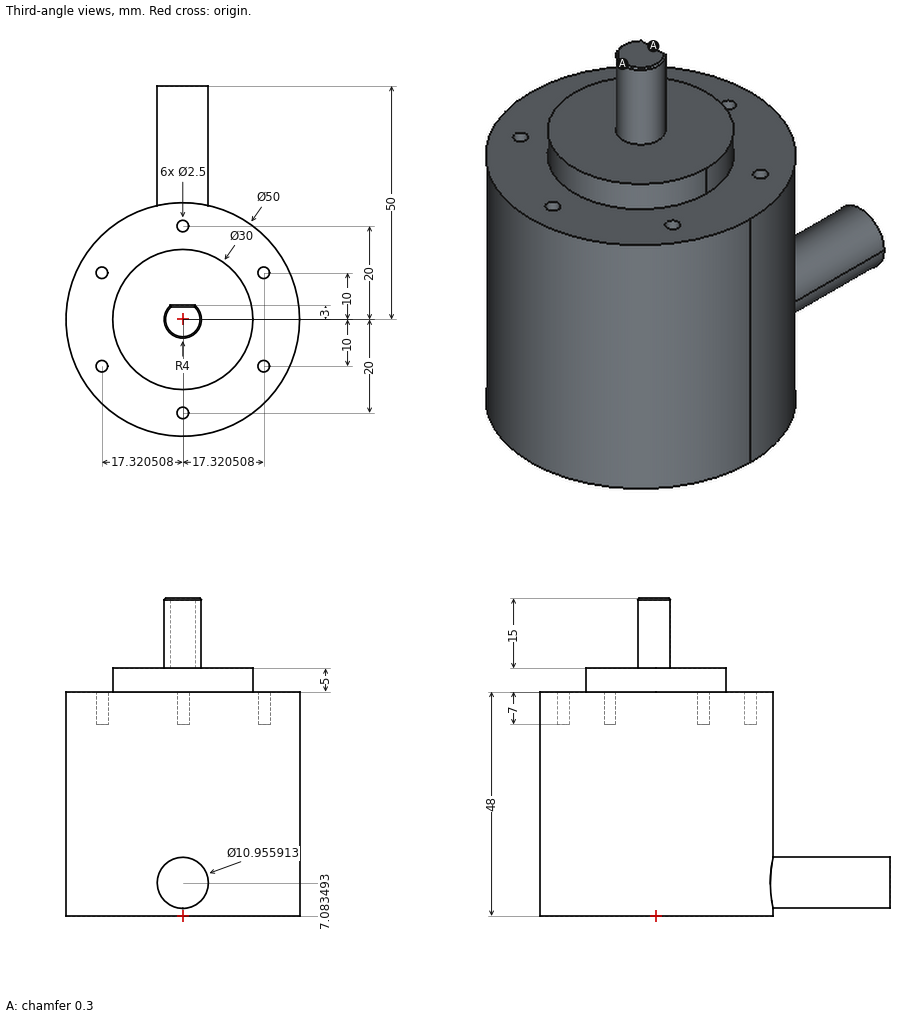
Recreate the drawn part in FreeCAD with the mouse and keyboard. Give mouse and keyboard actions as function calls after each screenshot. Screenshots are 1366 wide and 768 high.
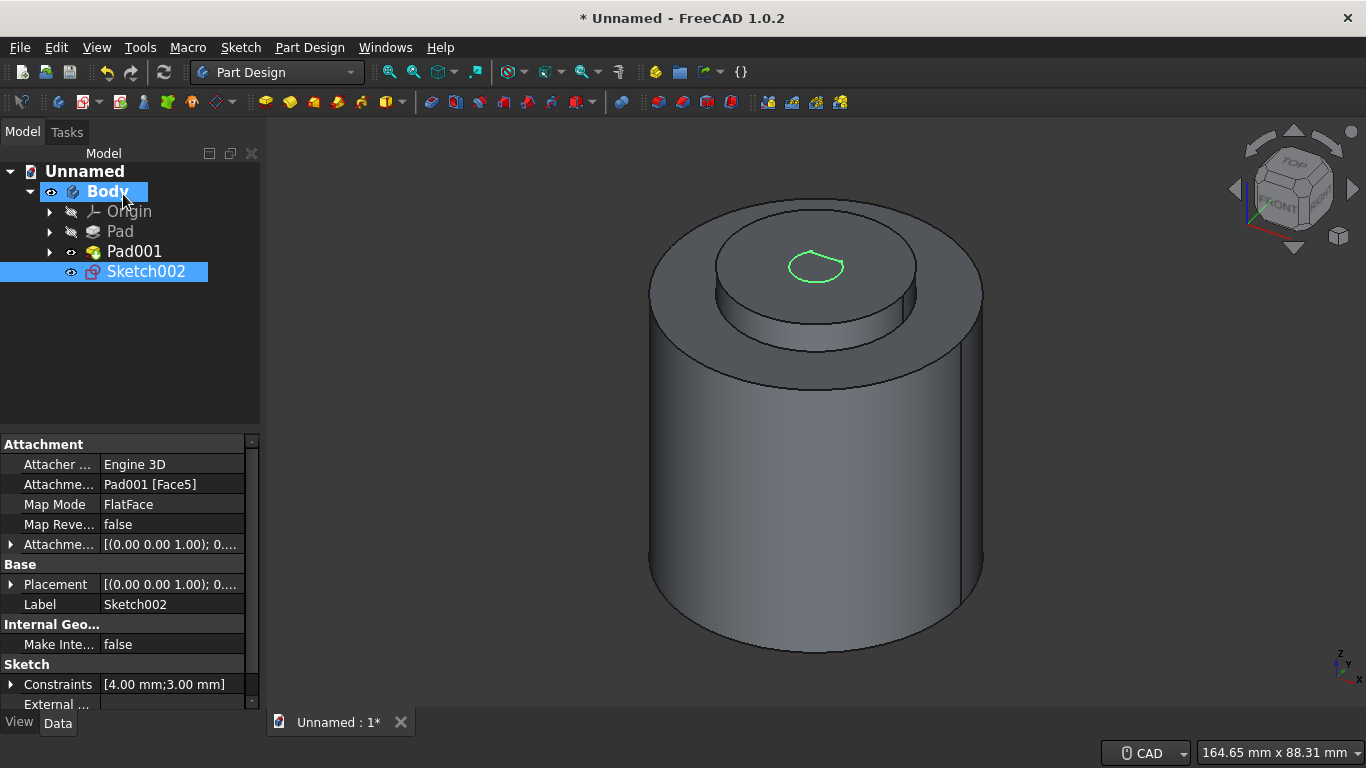
click(266, 102)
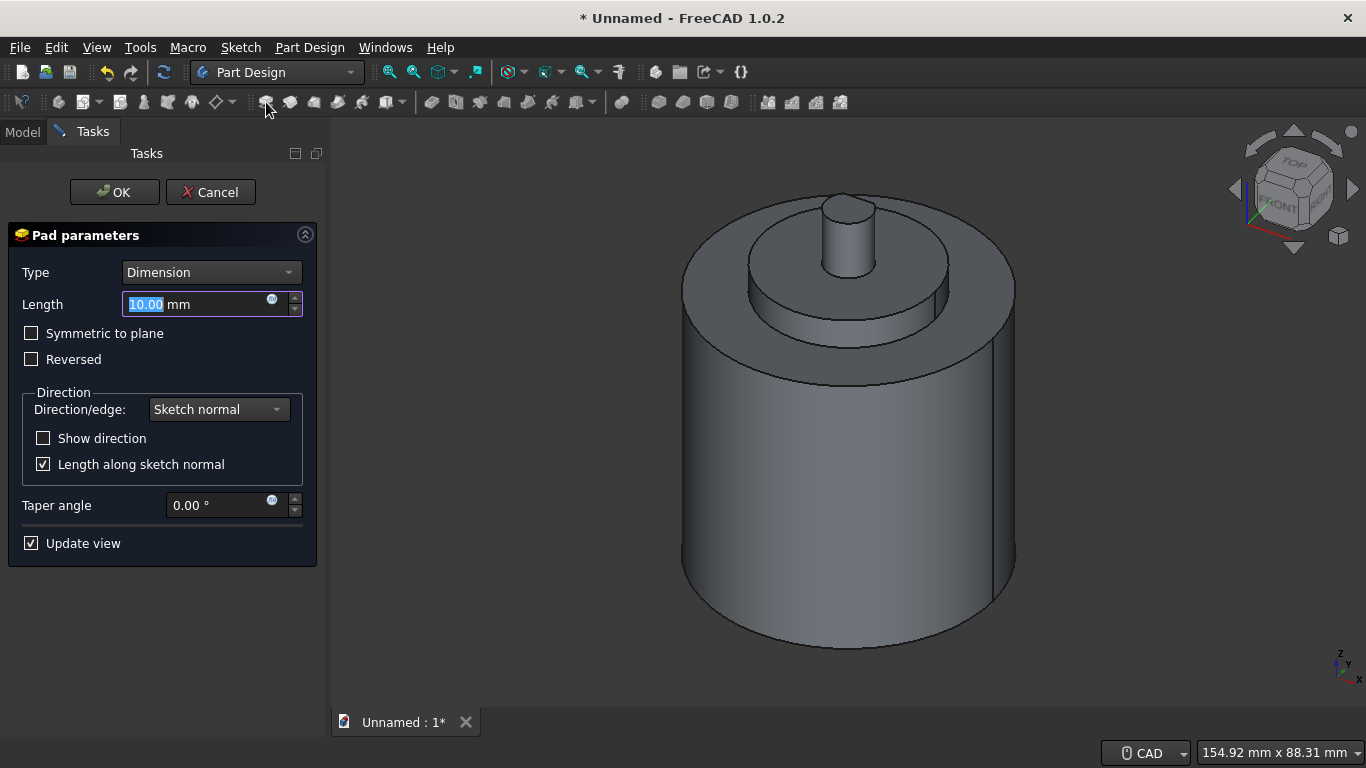
text(15)
key(Tab)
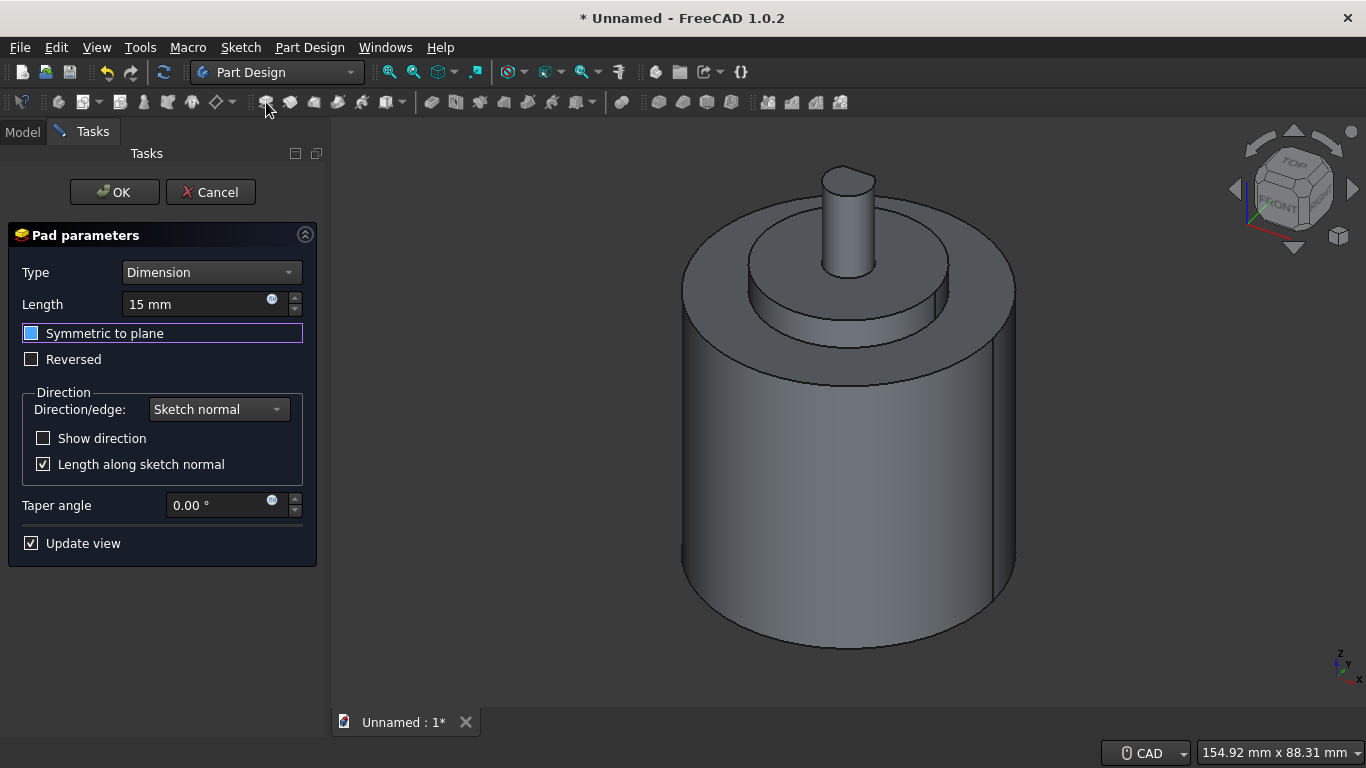
click(115, 192)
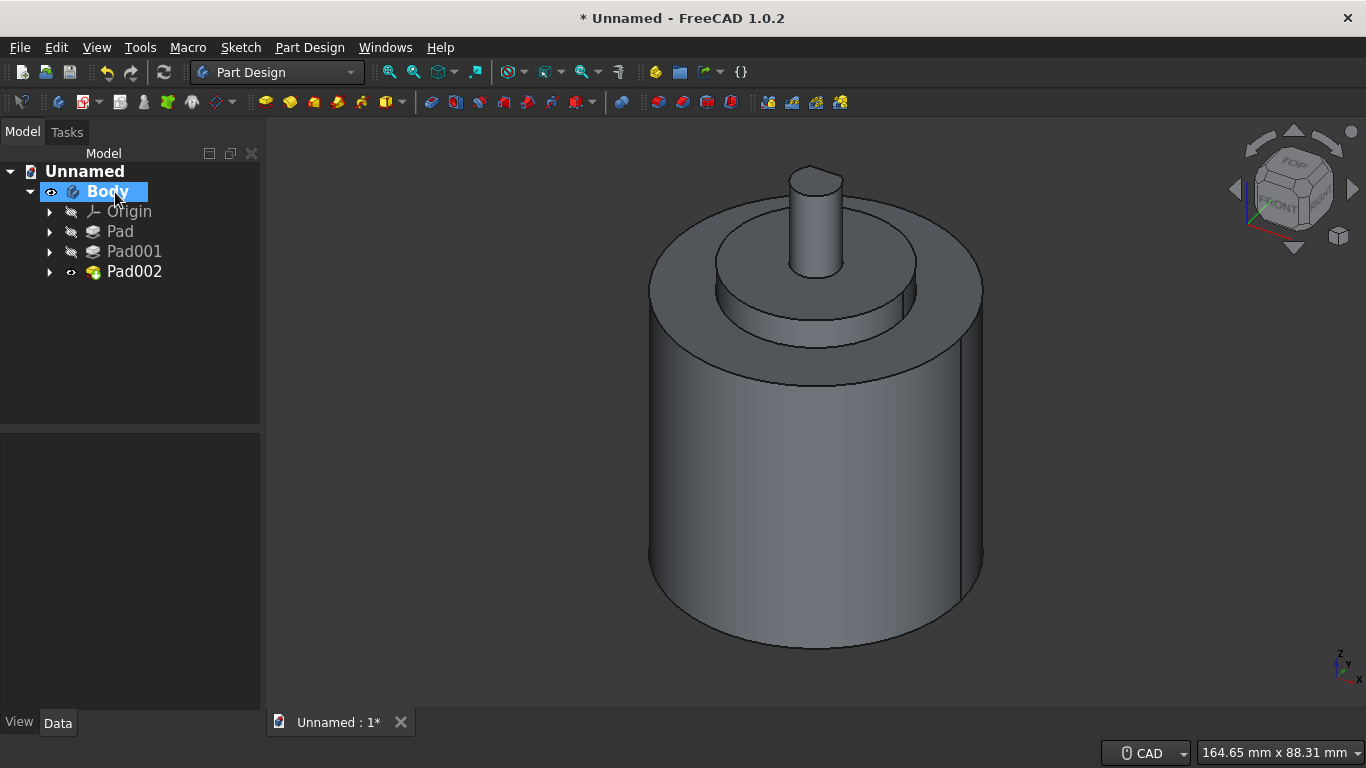
click(390, 72)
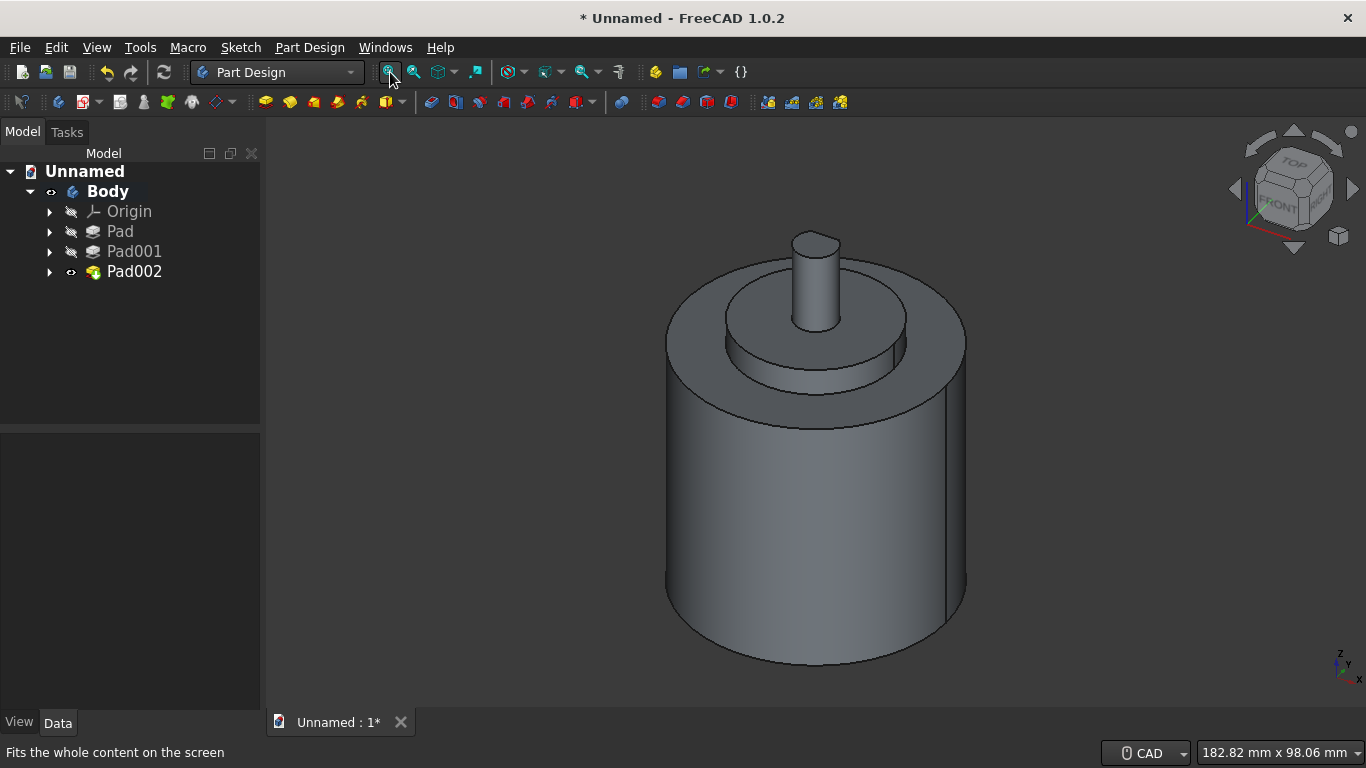
click(804, 255)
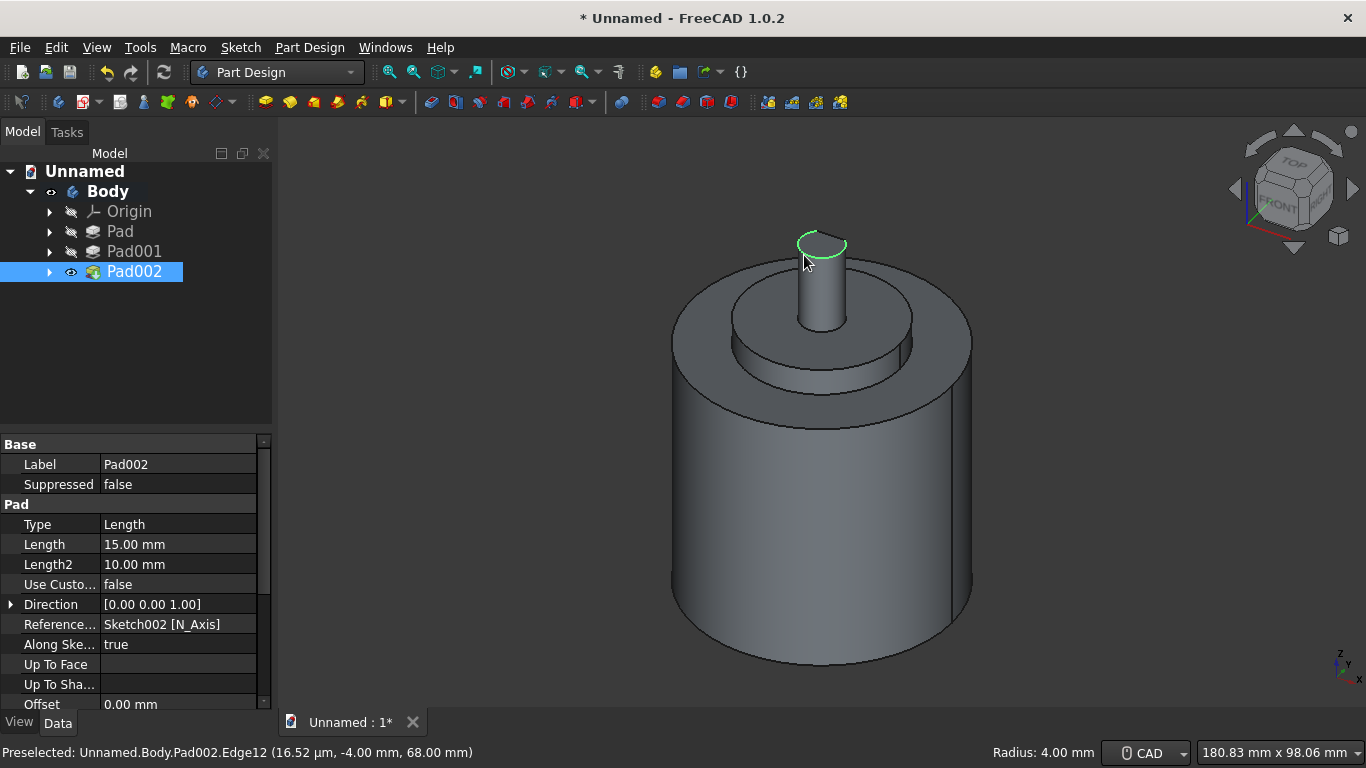
key(0)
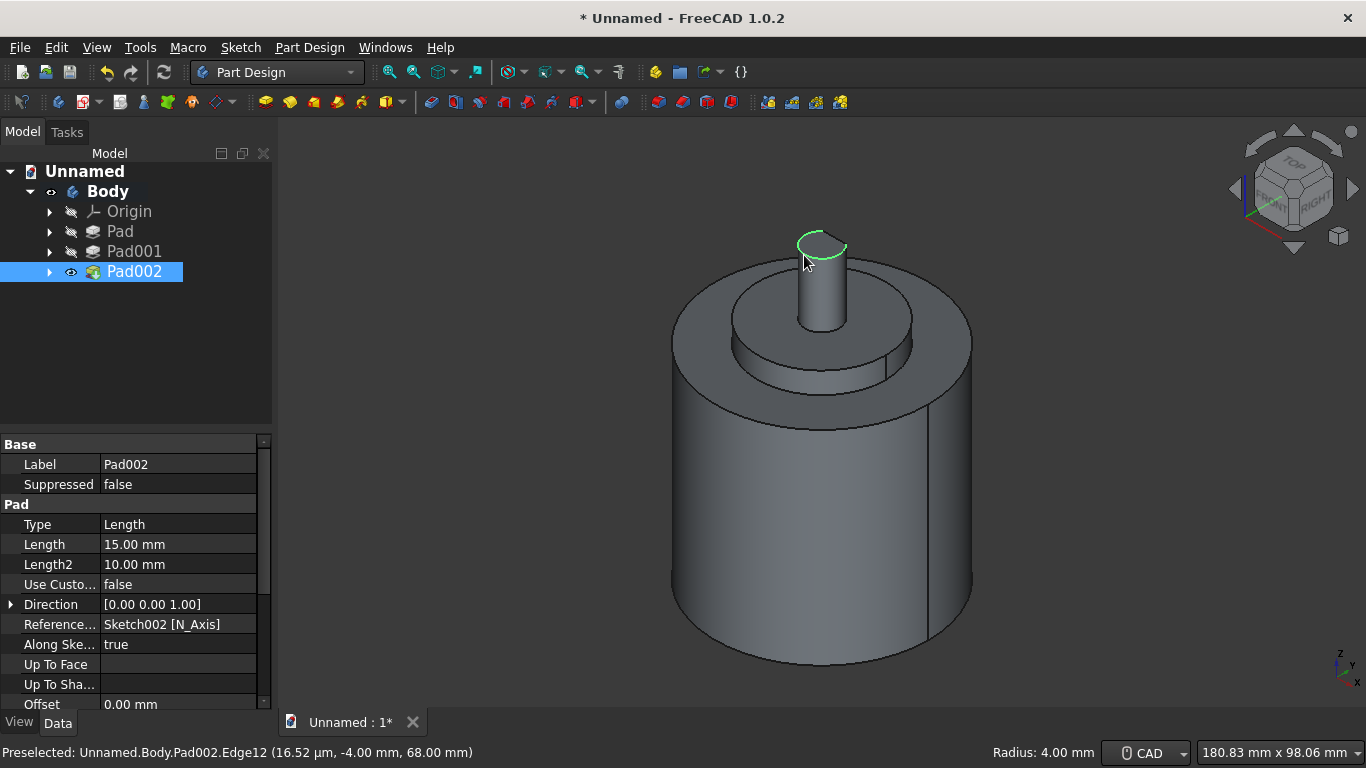
key(2)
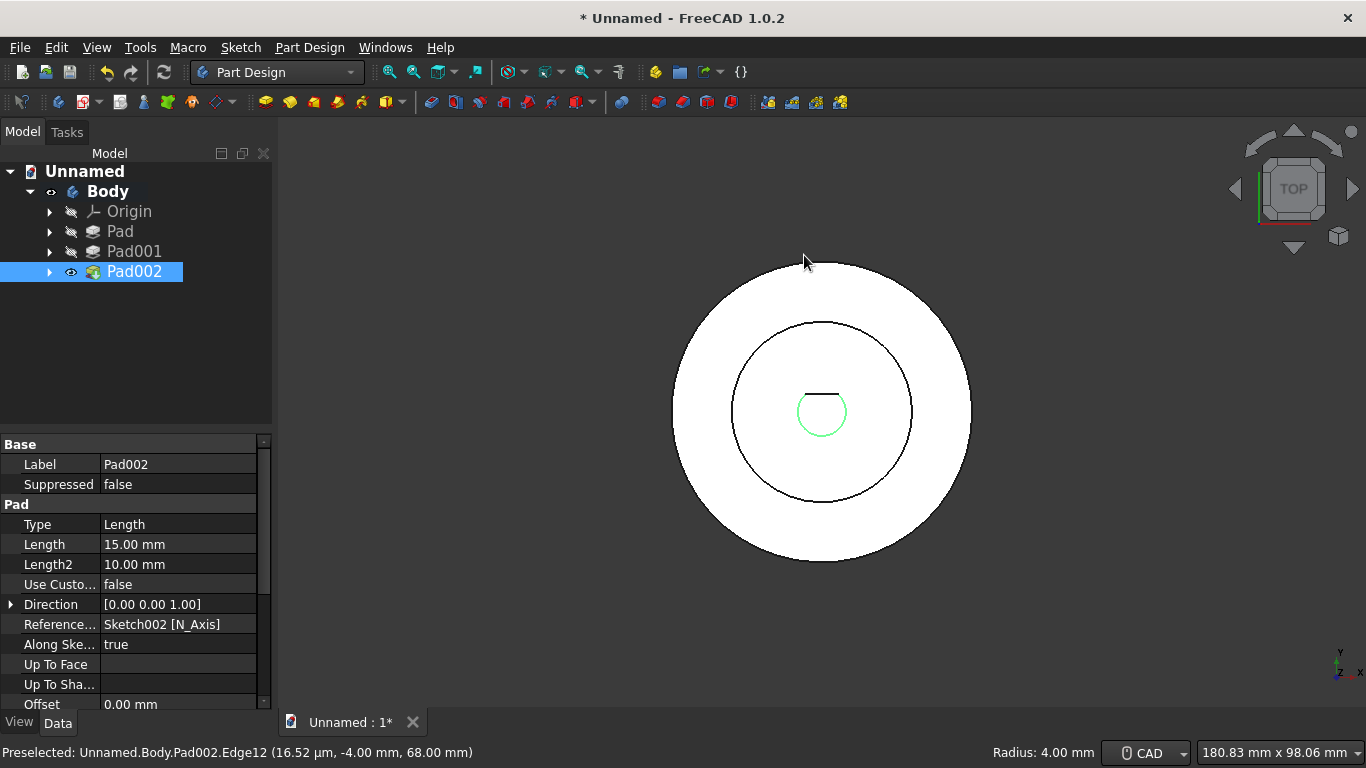
click(822, 393, ctrl)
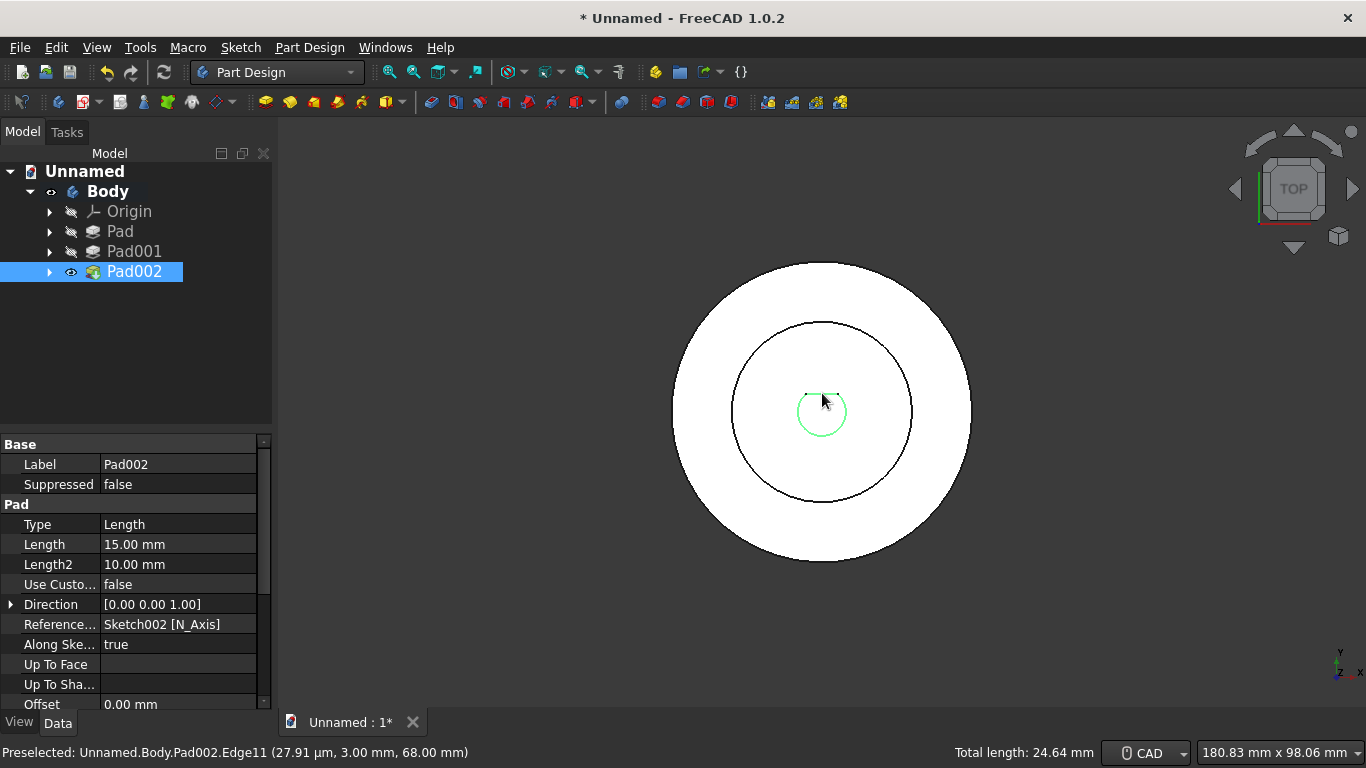
click(684, 102)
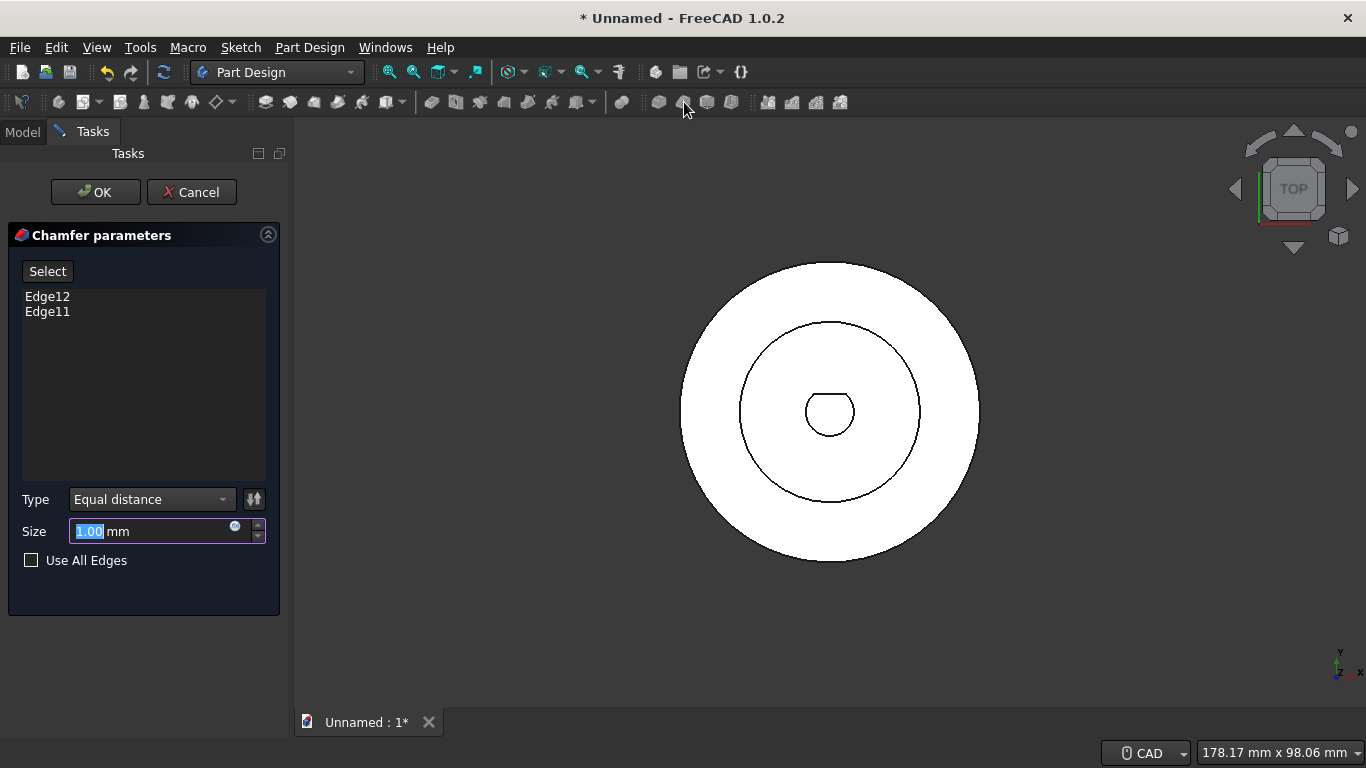
text(0.3)
key(Tab)